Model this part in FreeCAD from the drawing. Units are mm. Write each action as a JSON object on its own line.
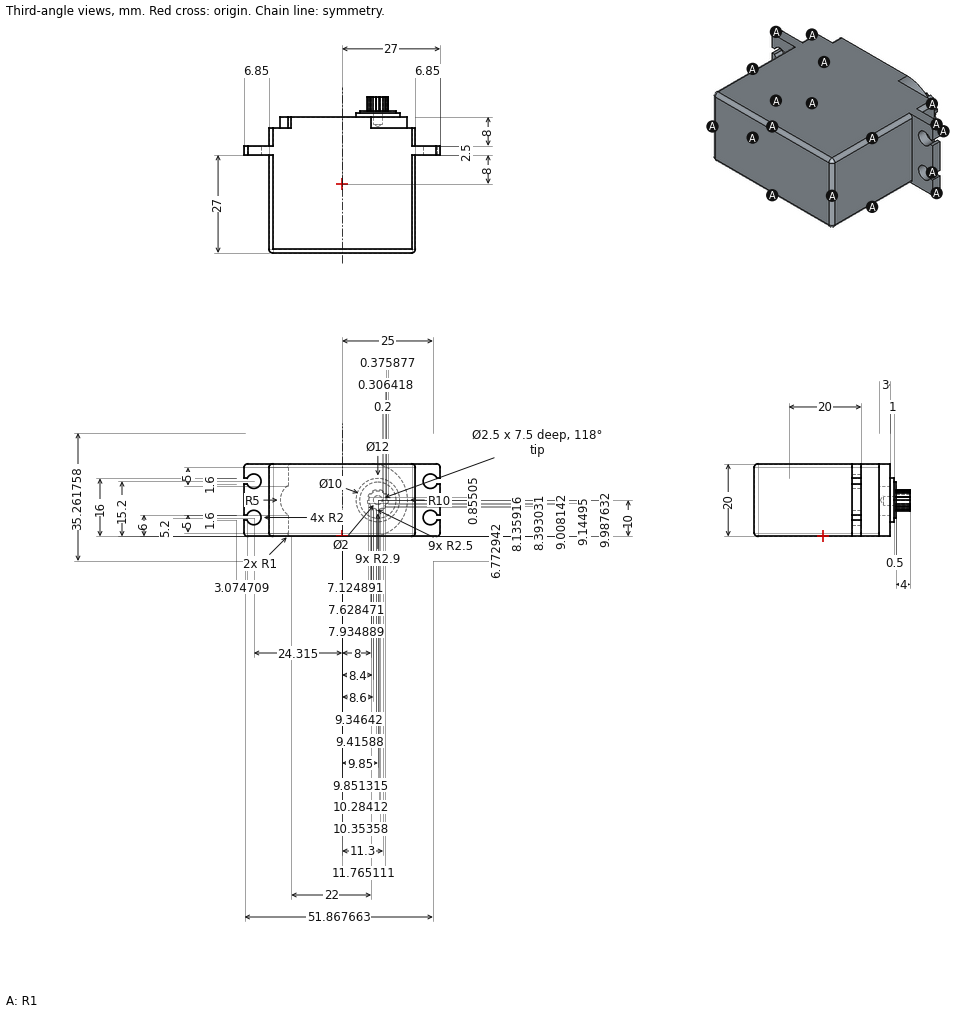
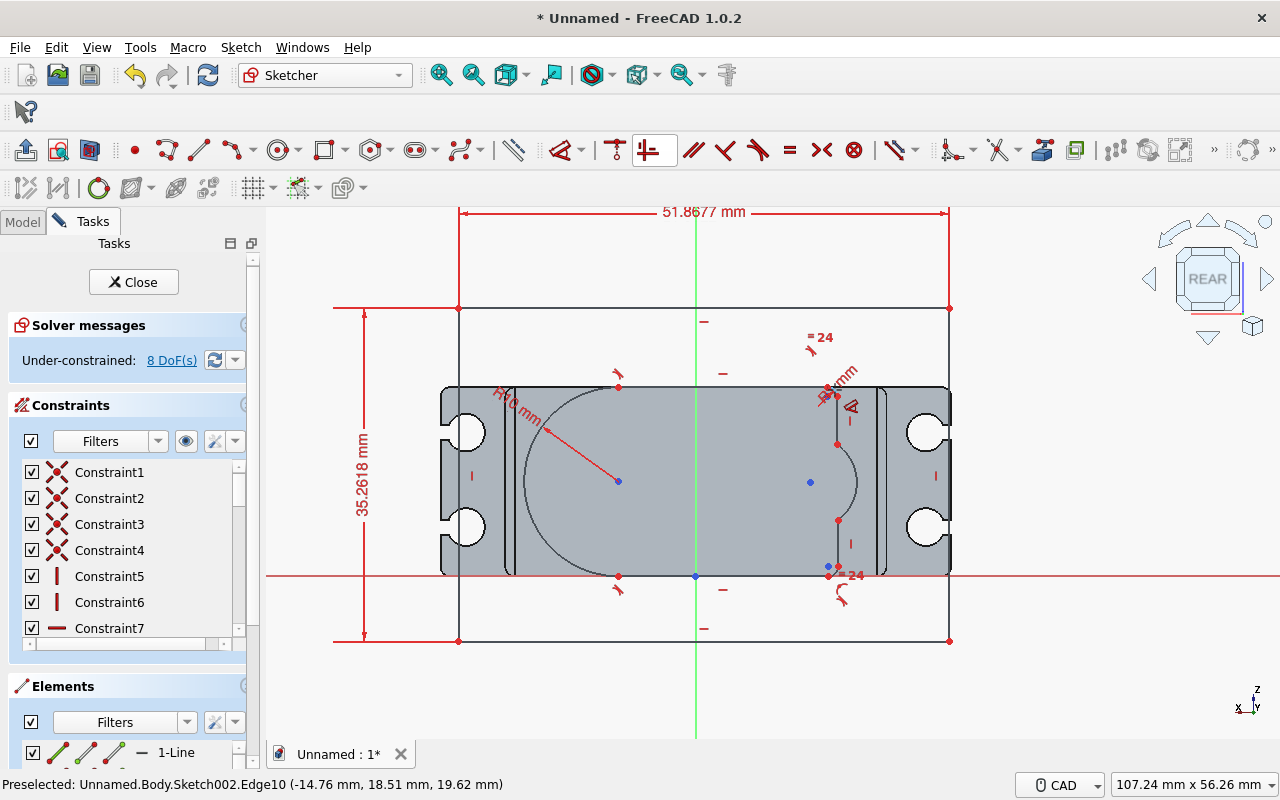
{"action": "left_click", "coordinate": [854, 499]}
{"action": "left_click", "coordinate": [884, 510]}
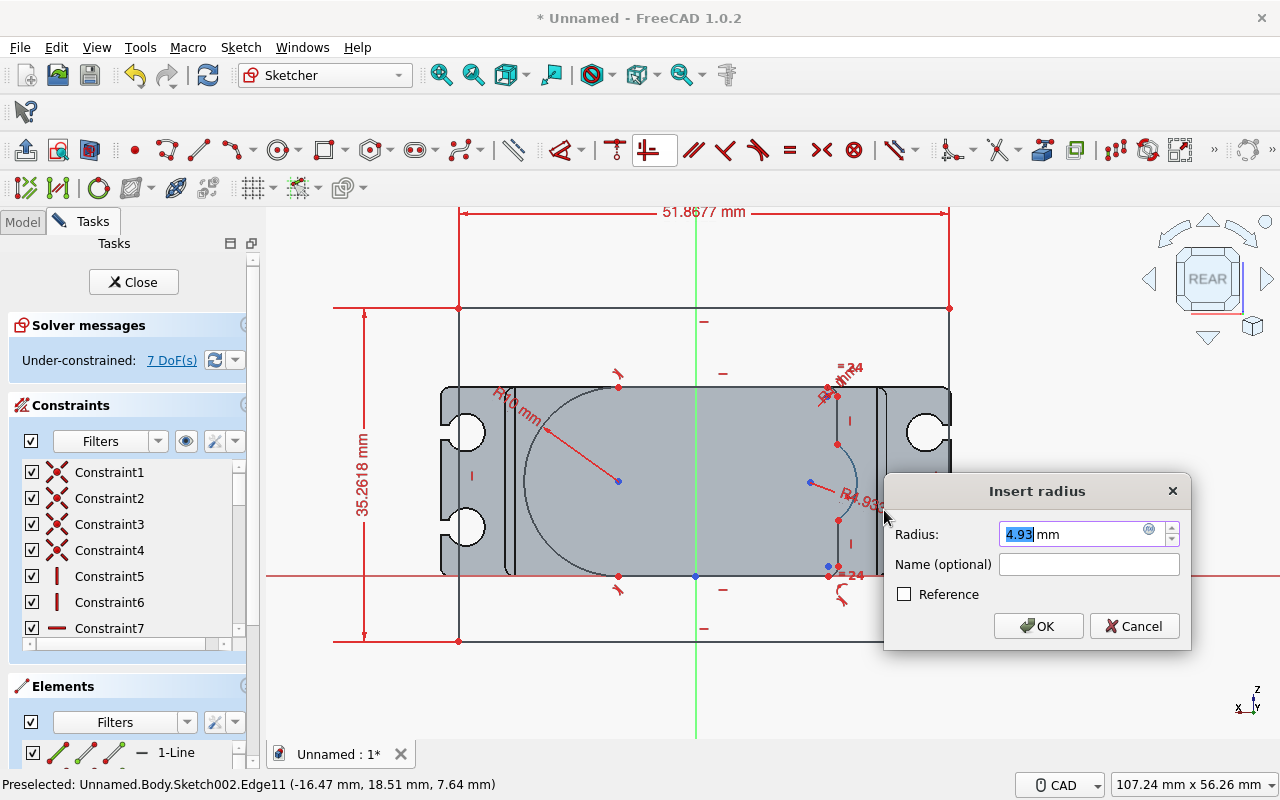
{"action": "type", "text": "5"}
{"action": "key", "text": "Return"}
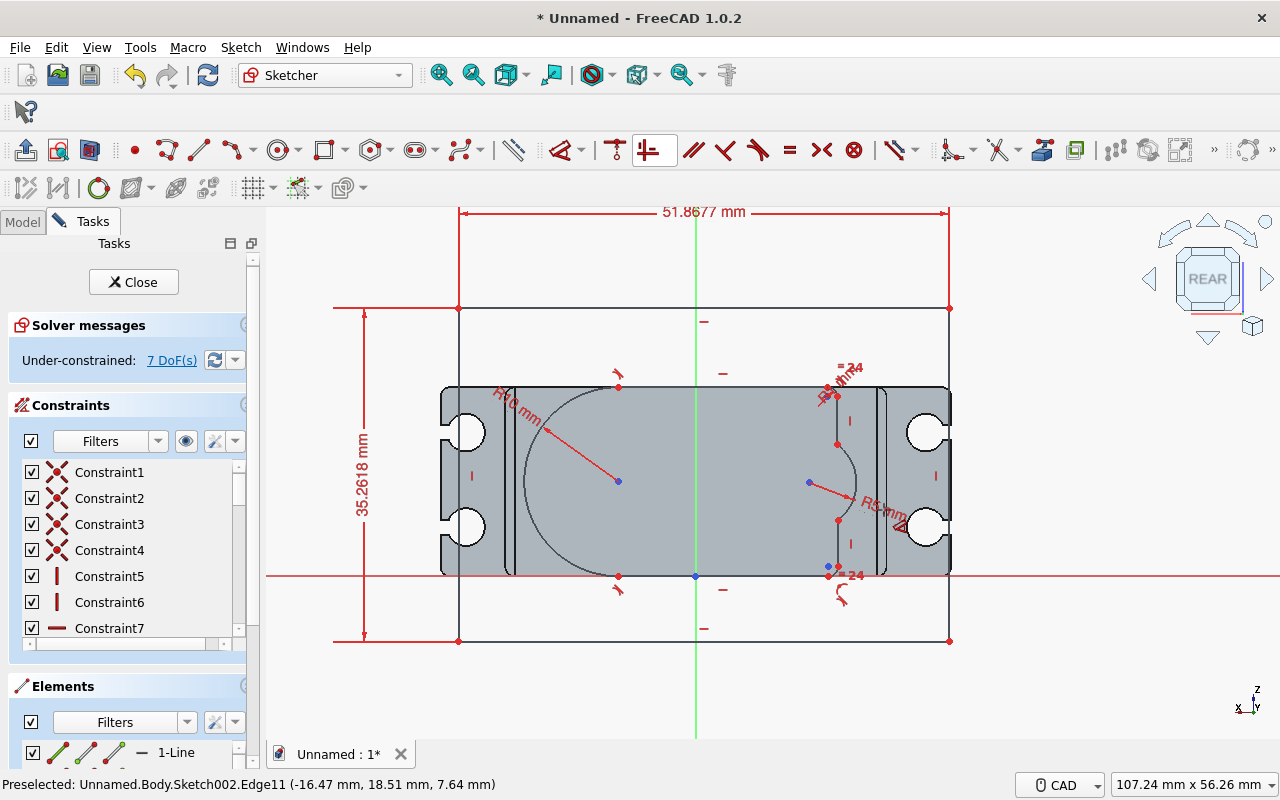
{"action": "left_click", "coordinate": [837, 411]}
{"action": "left_click", "coordinate": [871, 421]}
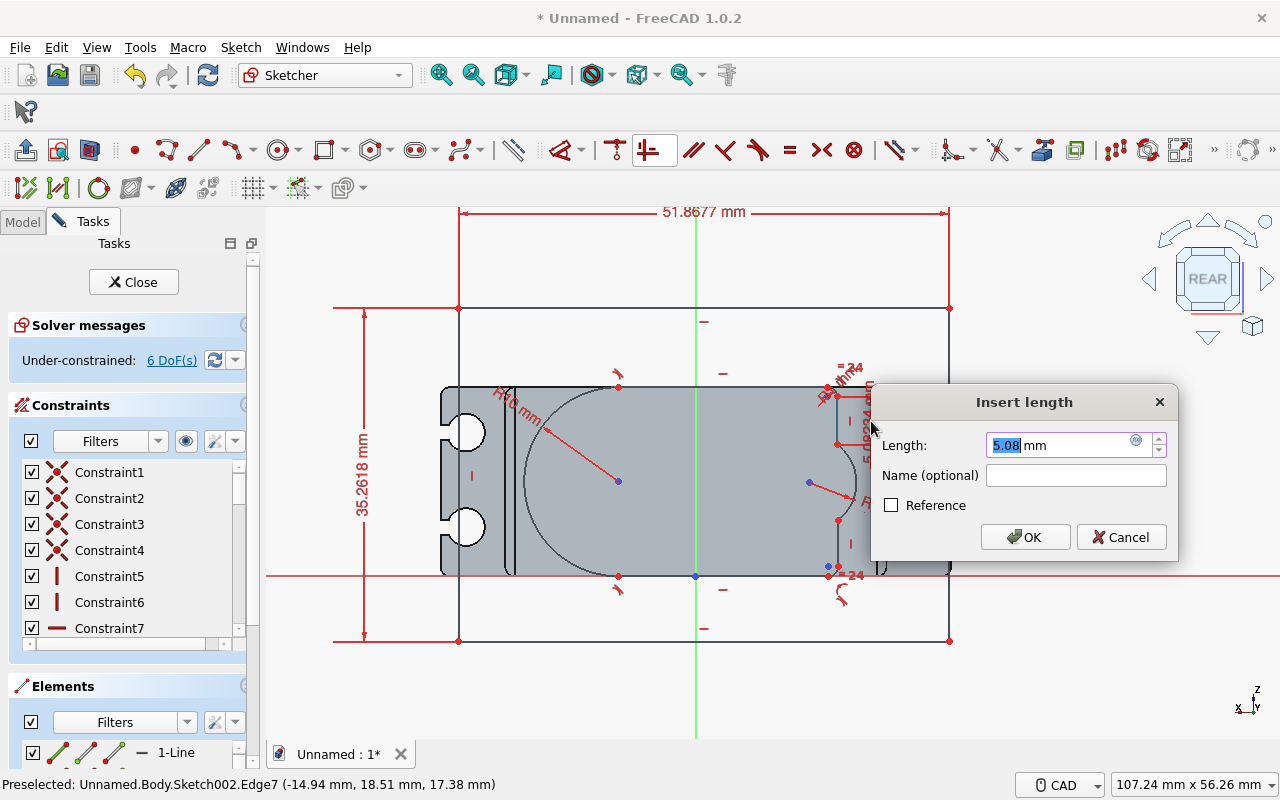
{"action": "type", "text": "5"}
{"action": "key", "text": "Return"}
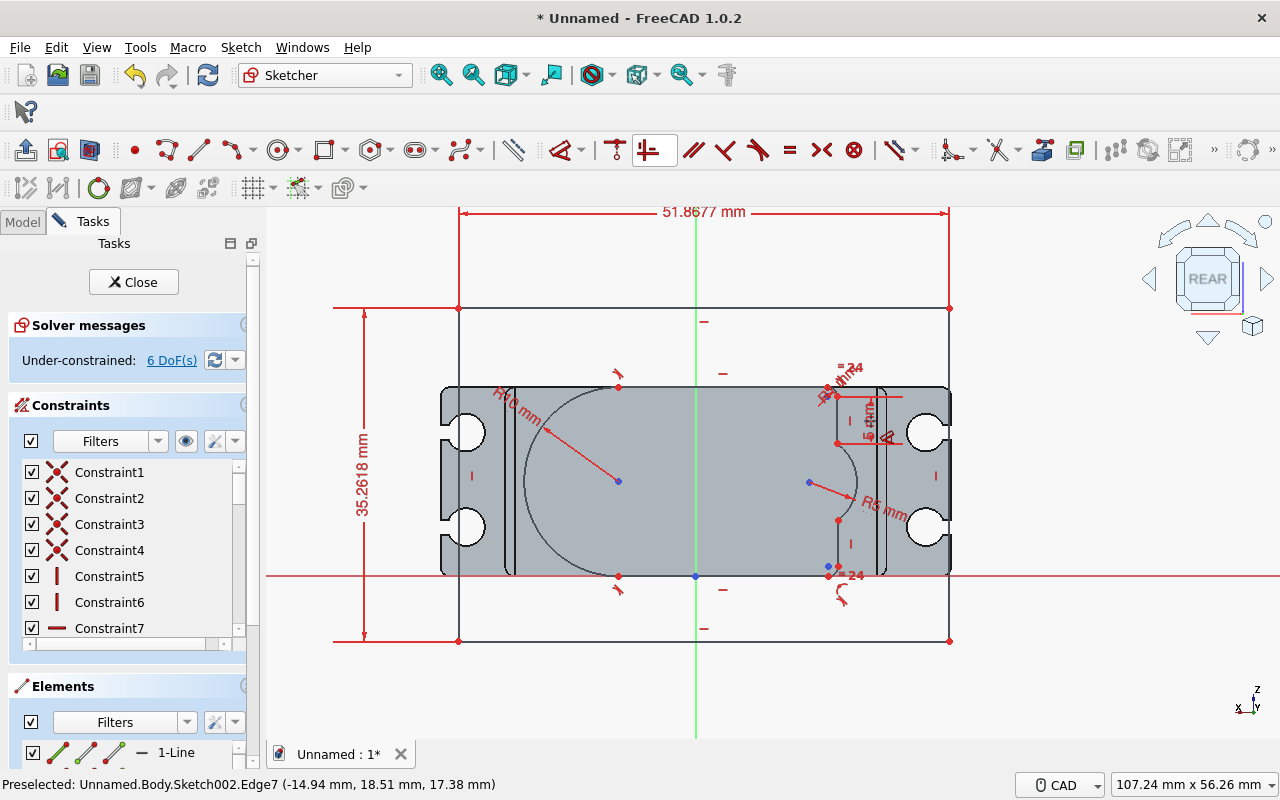
{"action": "left_click", "coordinate": [838, 534]}
{"action": "left_click", "coordinate": [872, 543]}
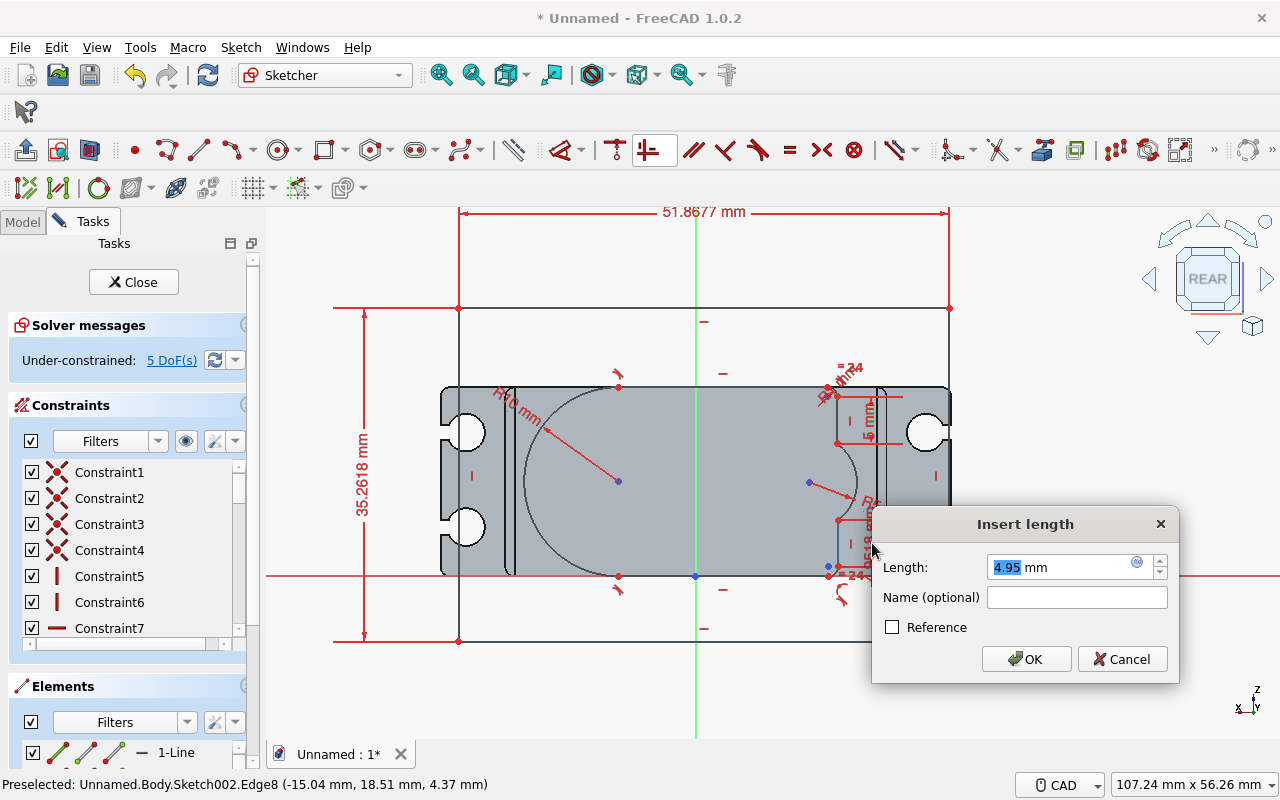
{"action": "type", "text": "5"}
{"action": "key", "text": "Return"}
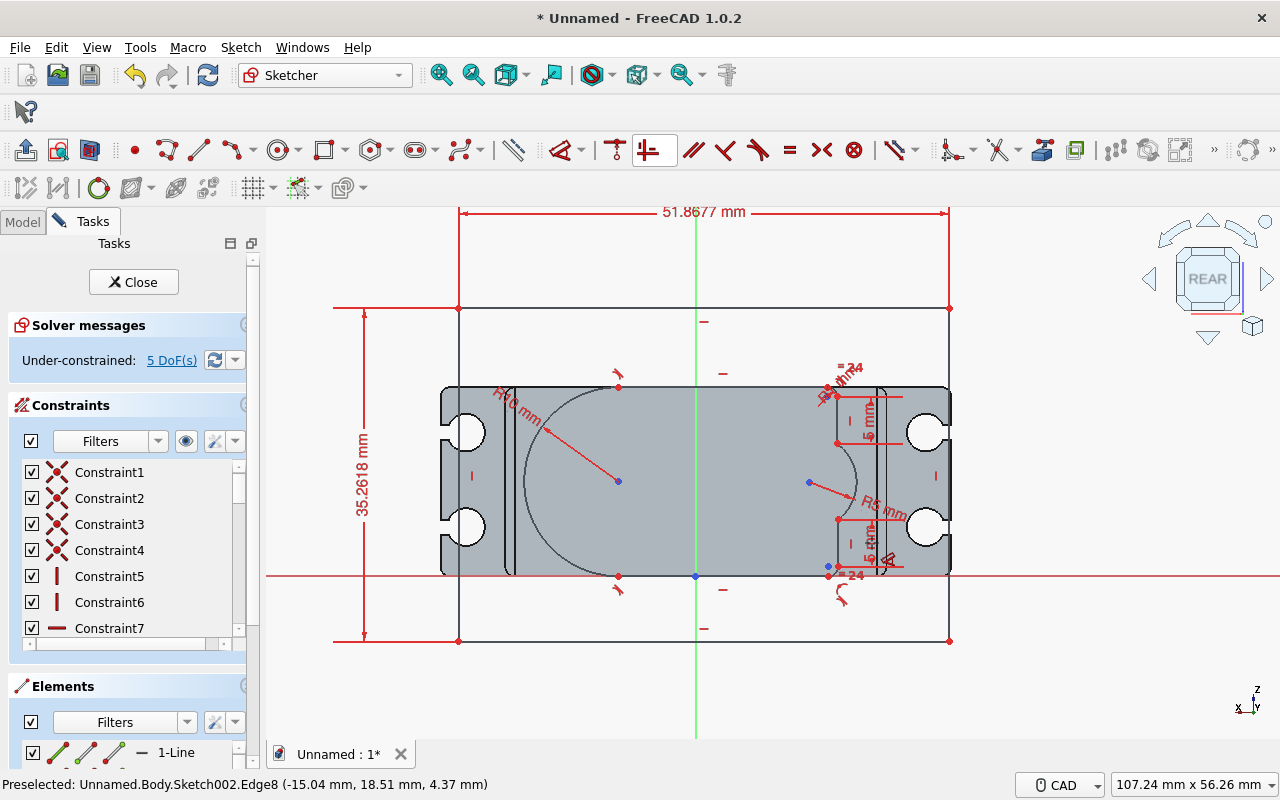
{"action": "left_click", "coordinate": [766, 576]}
{"action": "left_click", "coordinate": [724, 610]}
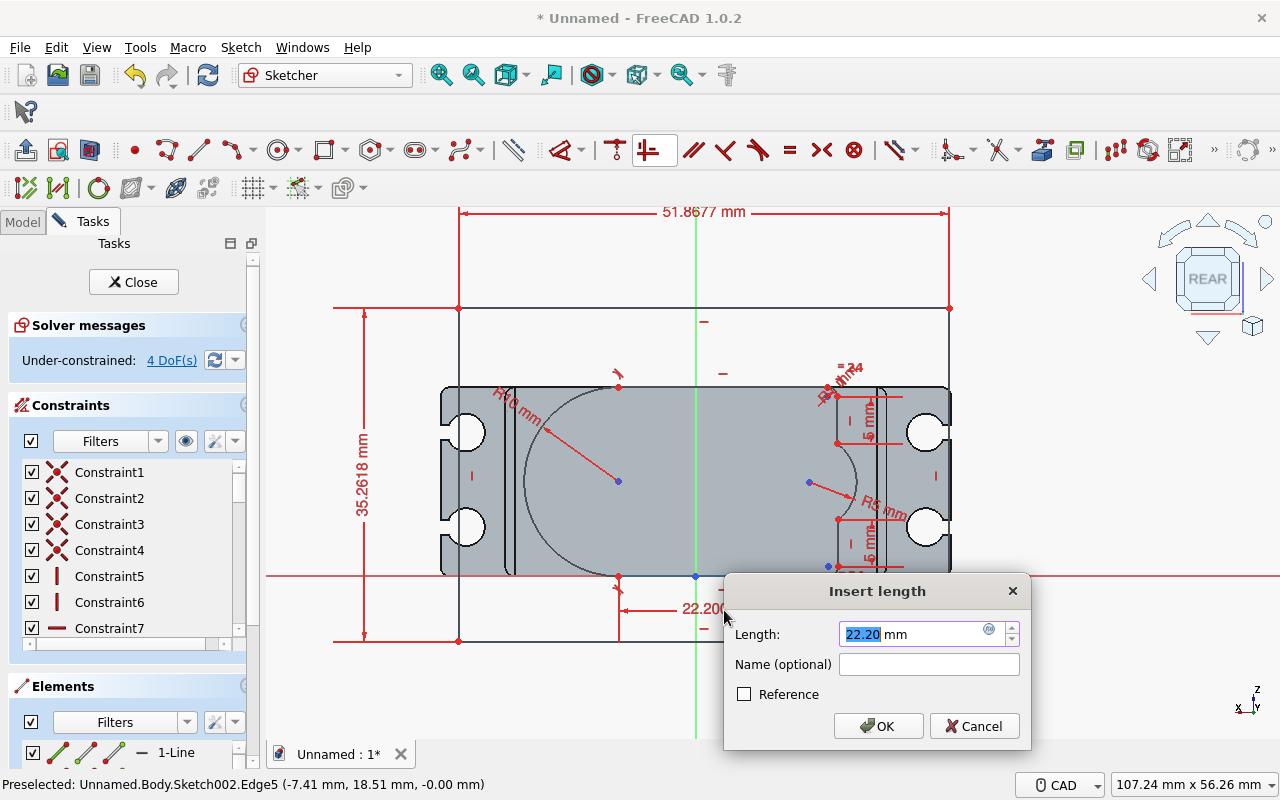
{"action": "type", "text": "22"}
{"action": "key", "text": "Return"}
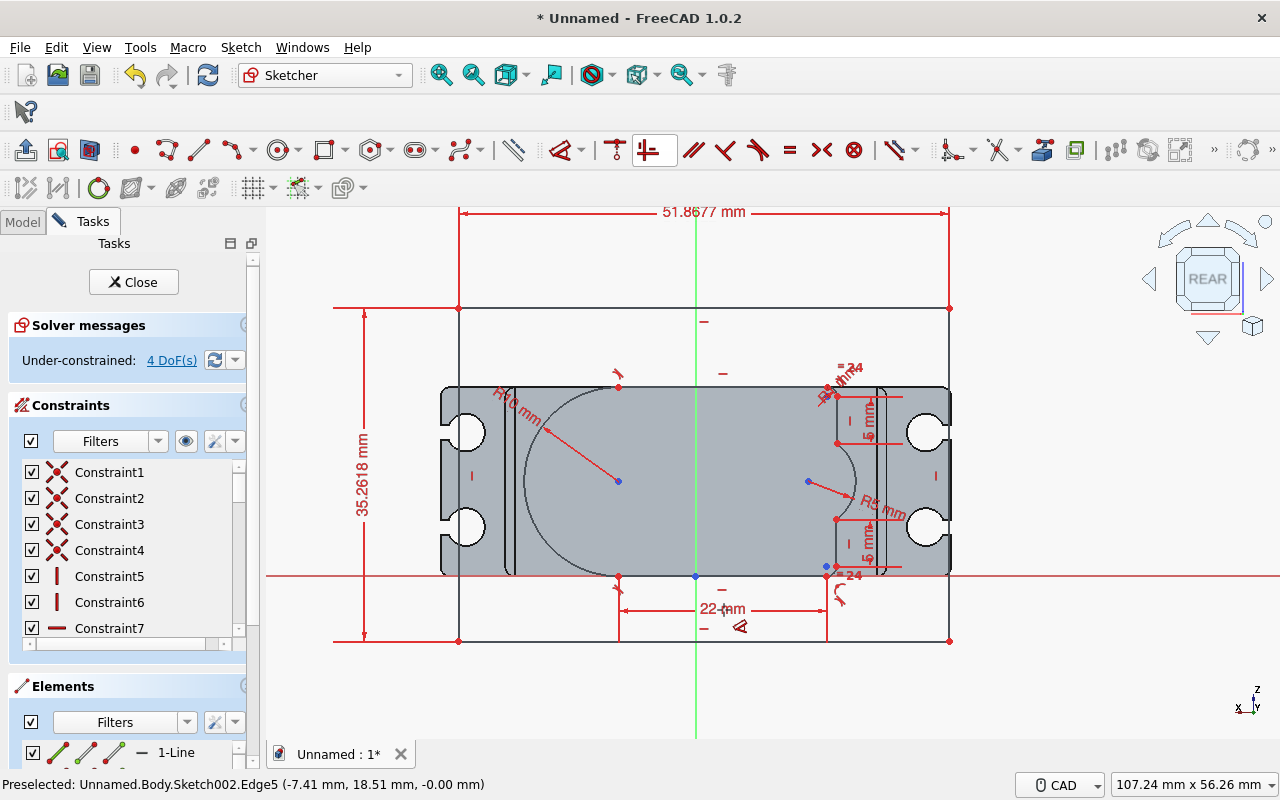
{"action": "left_click", "coordinate": [681, 387]}
{"action": "left_click", "coordinate": [723, 353]}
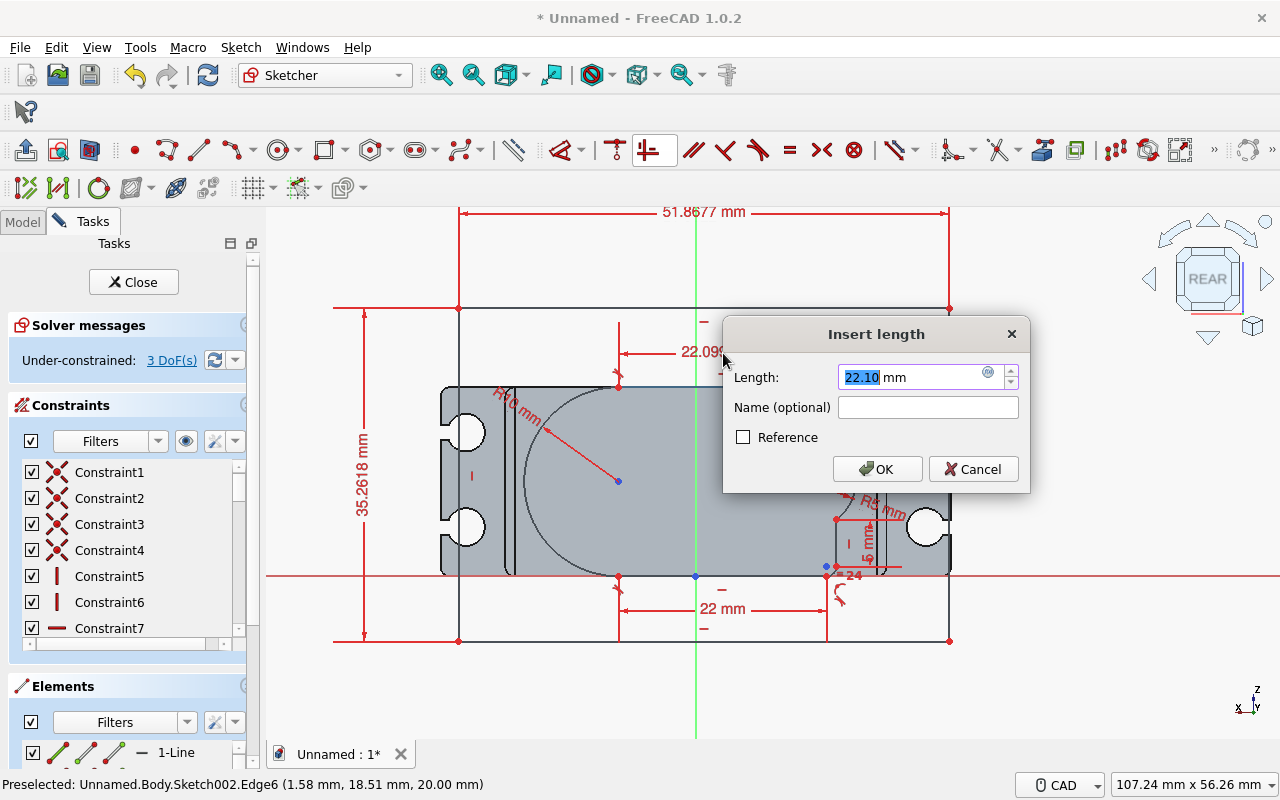
{"action": "type", "text": "22"}
{"action": "key", "text": "Return"}